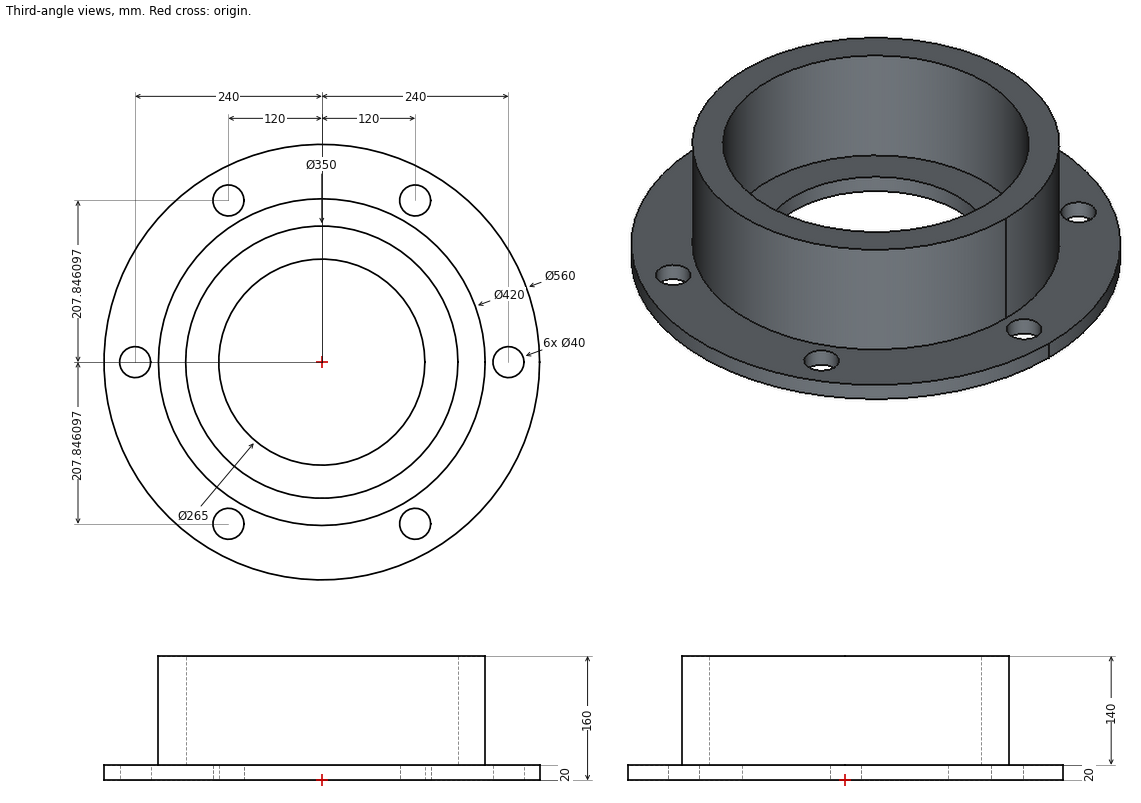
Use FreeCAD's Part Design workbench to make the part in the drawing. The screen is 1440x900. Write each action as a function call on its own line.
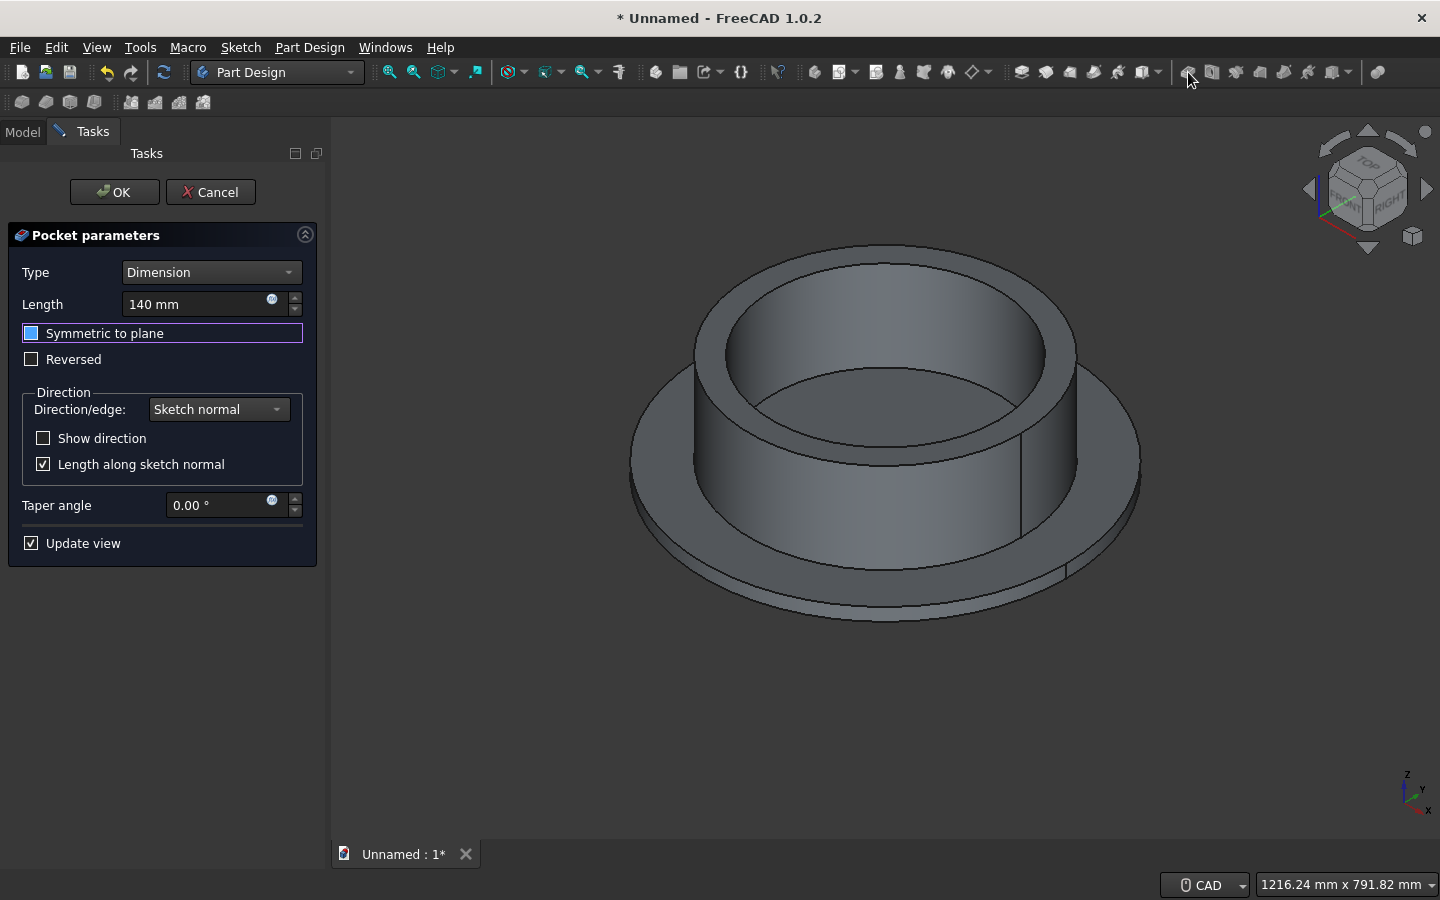
click(115, 192)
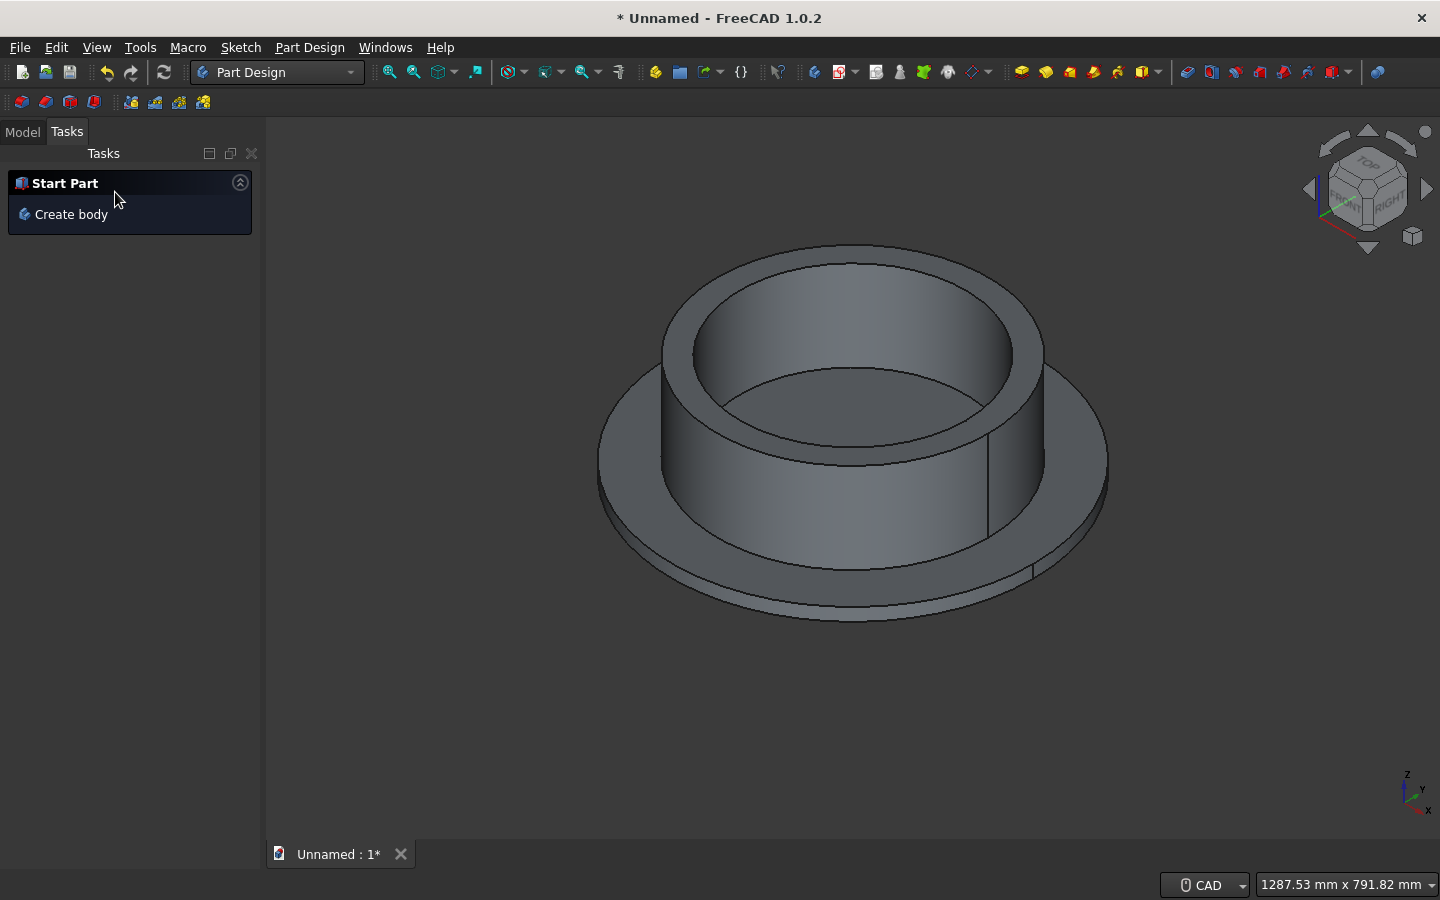
click(840, 72)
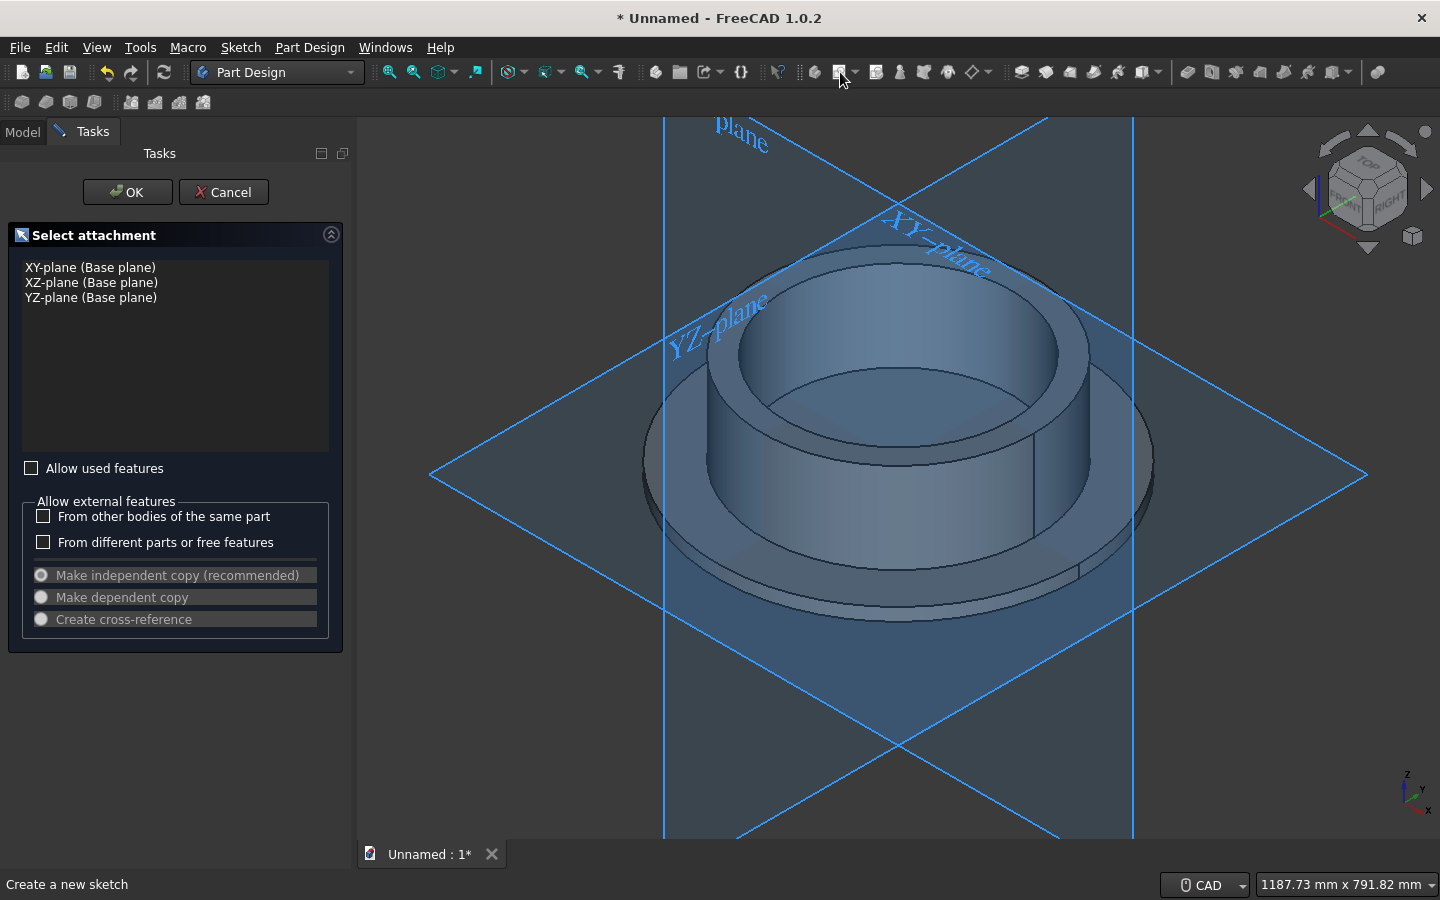
click(82, 268)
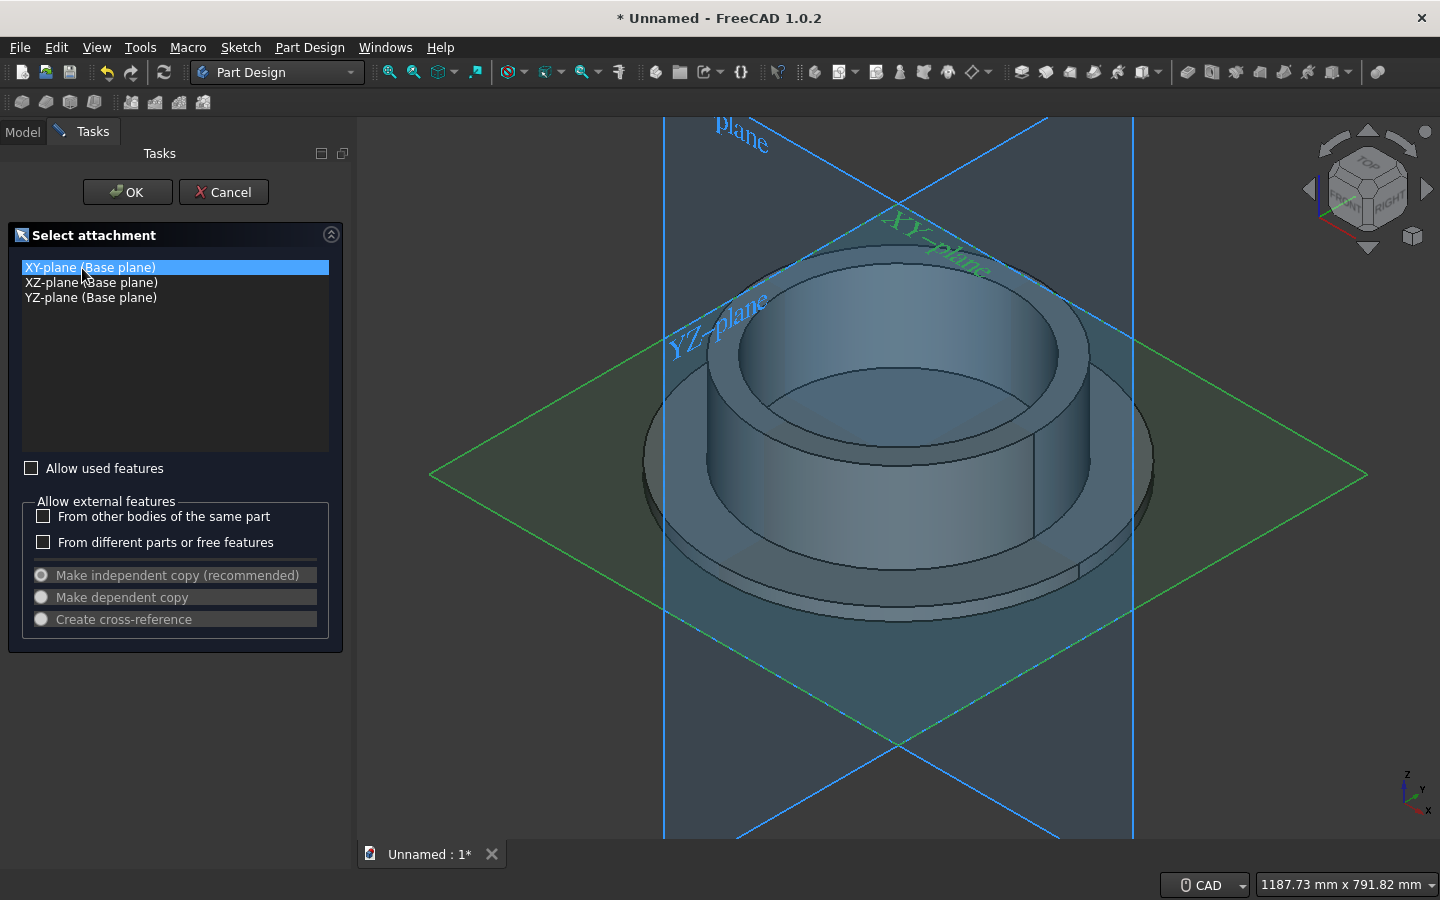
click(128, 192)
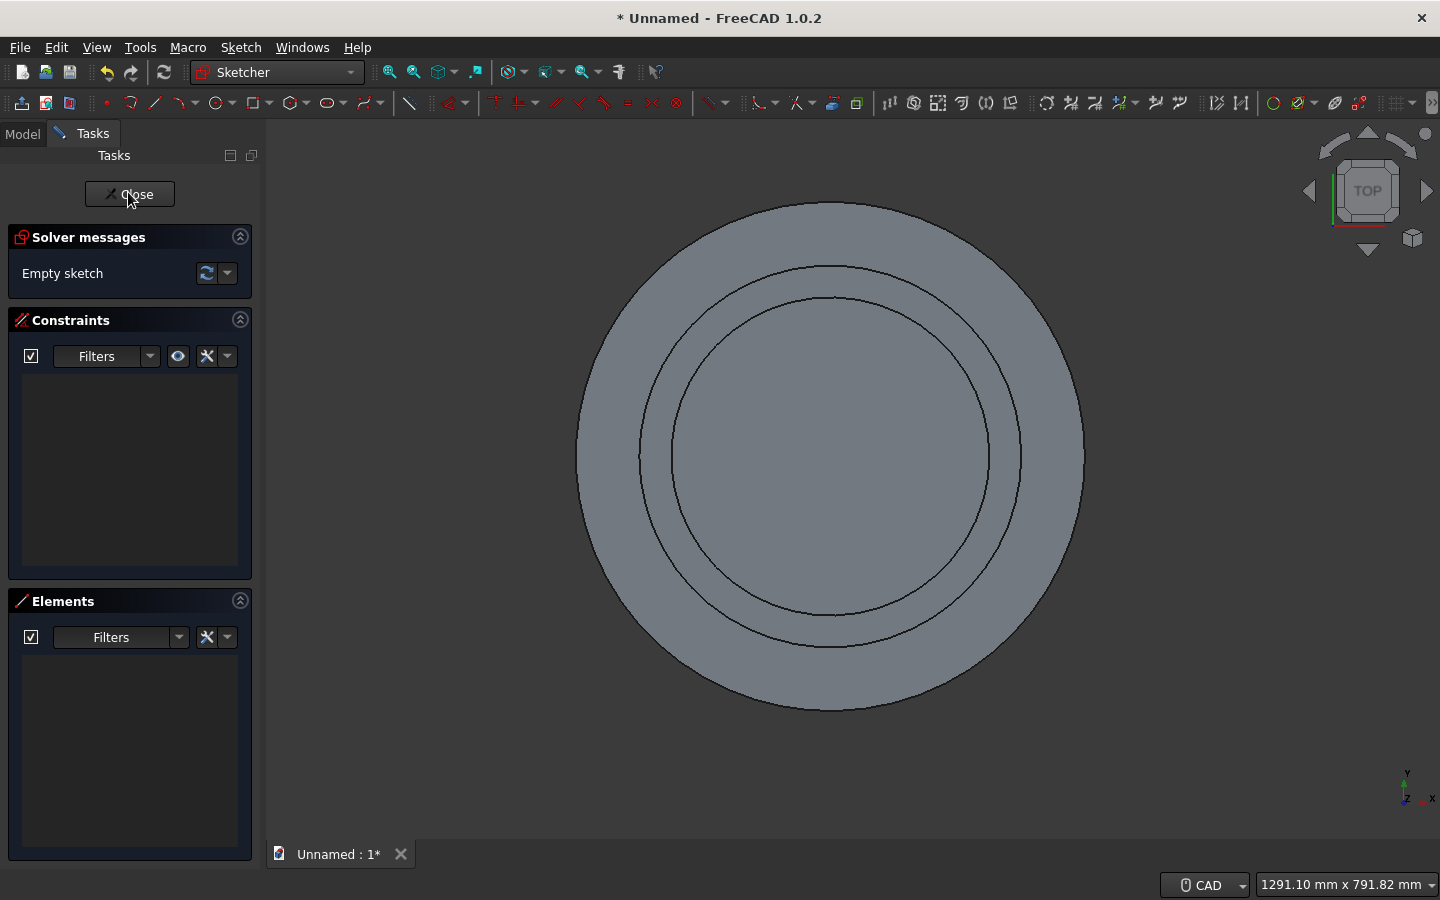
click(70, 104)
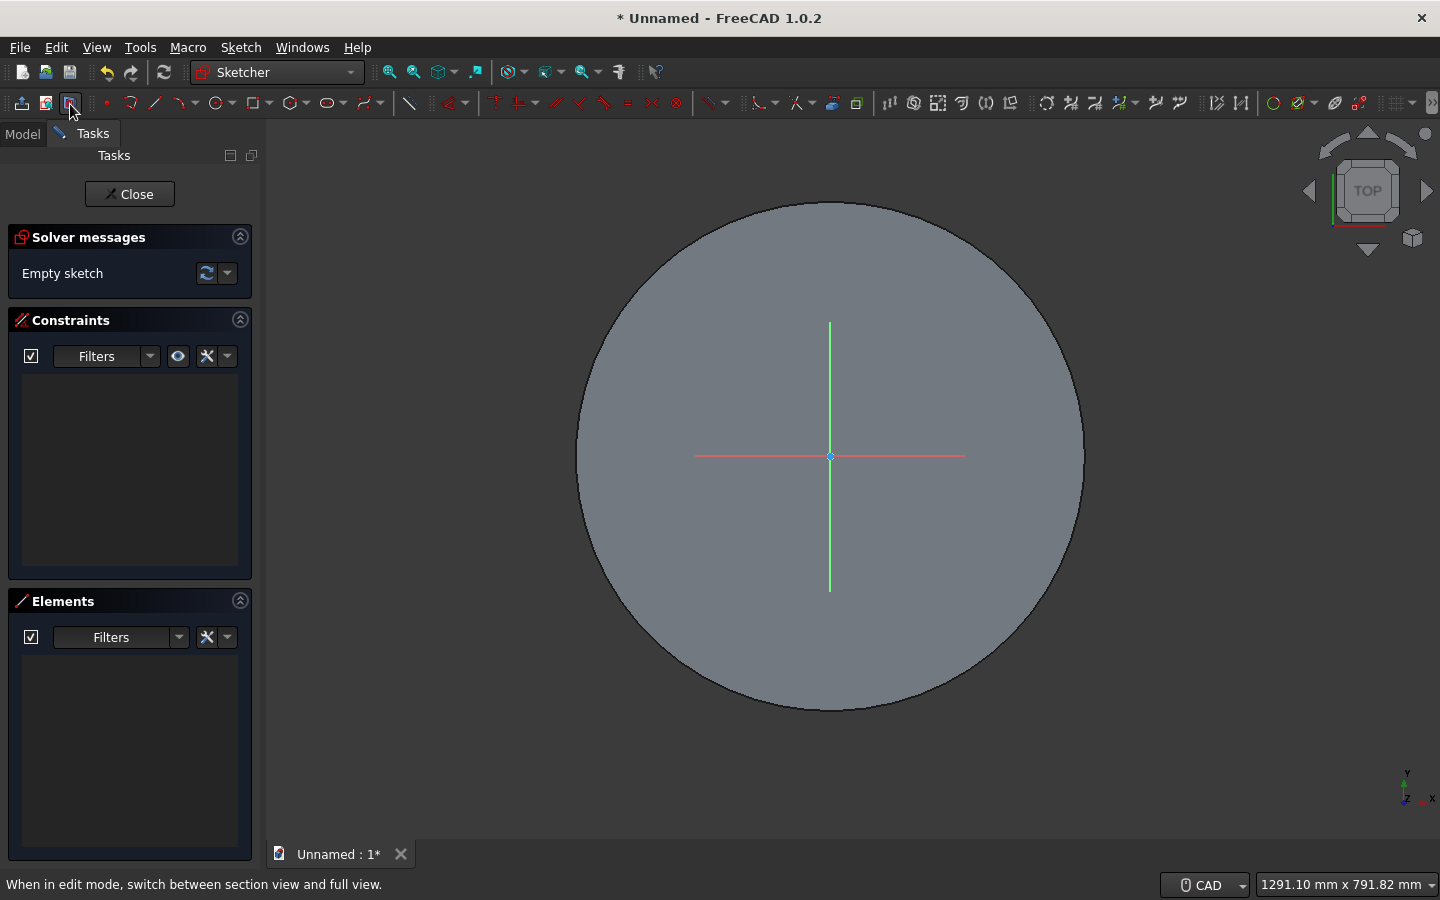
key(g)
key(c)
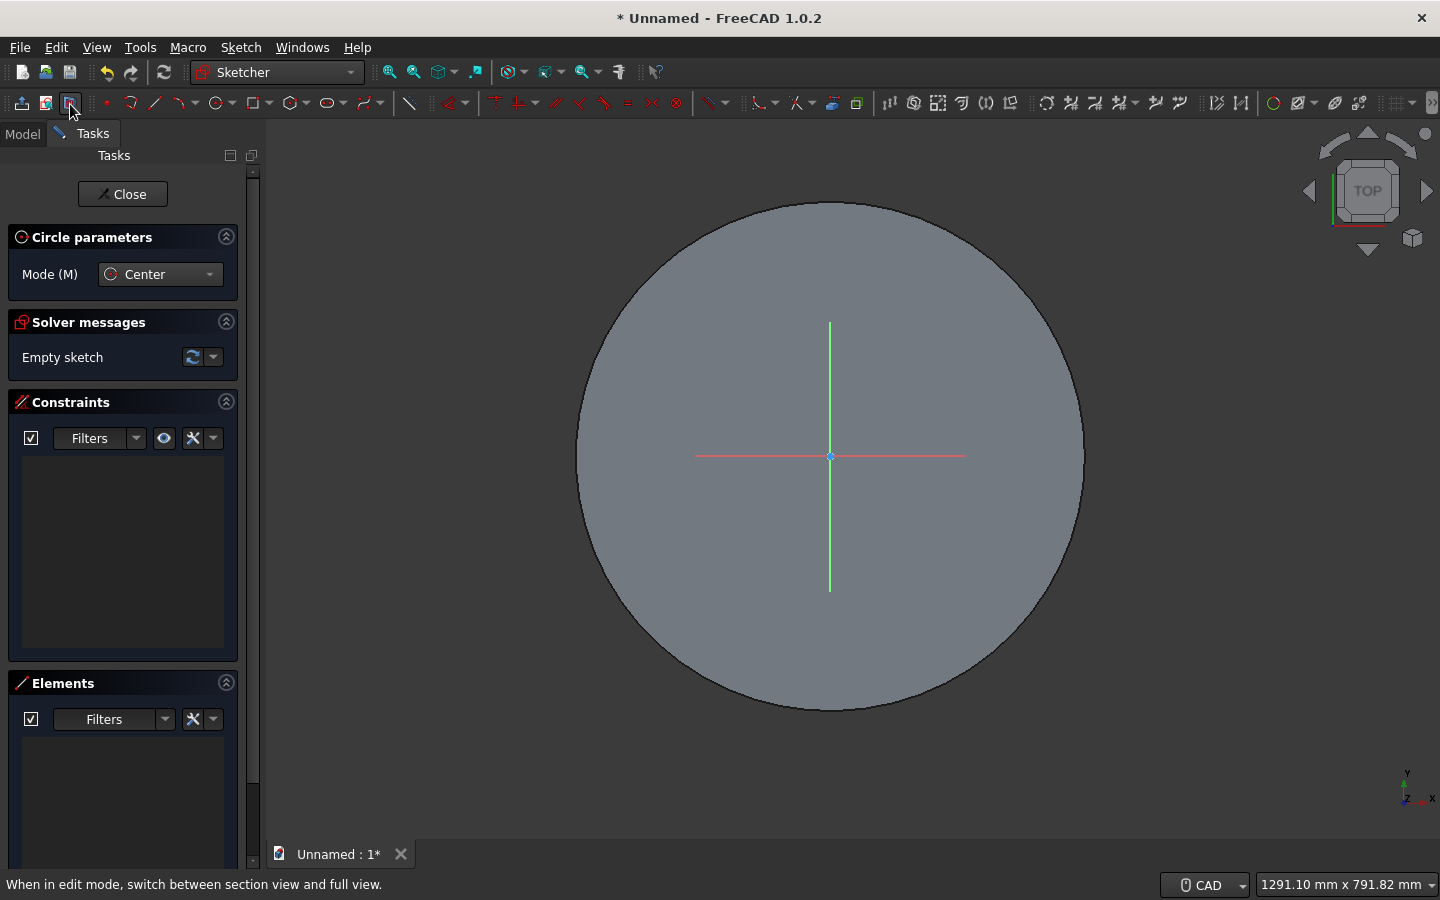
scroll(1049, 456, up, 2)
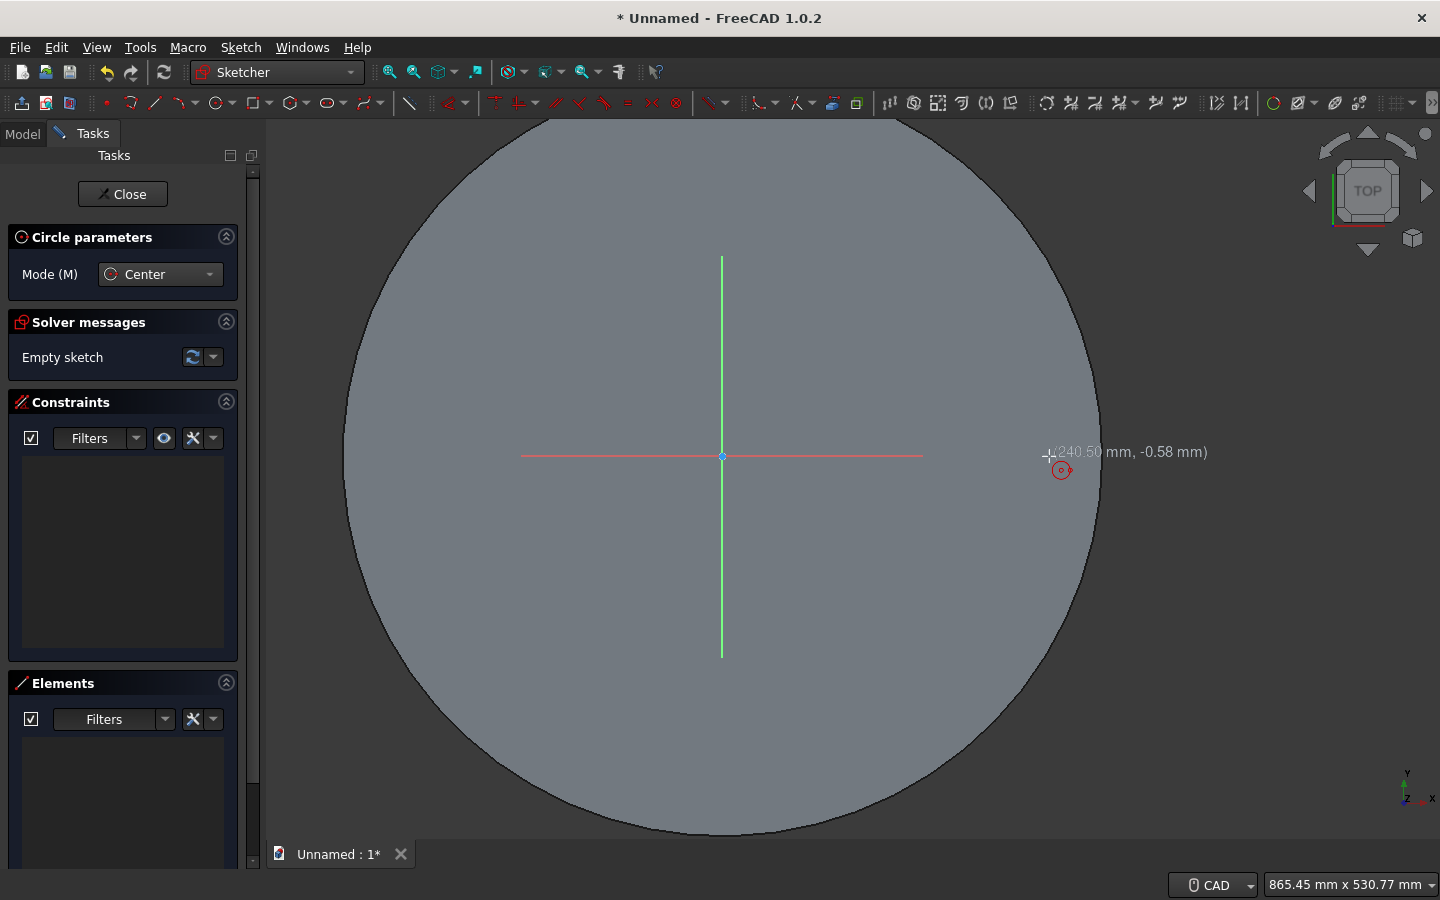
click(1048, 456)
click(1067, 437)